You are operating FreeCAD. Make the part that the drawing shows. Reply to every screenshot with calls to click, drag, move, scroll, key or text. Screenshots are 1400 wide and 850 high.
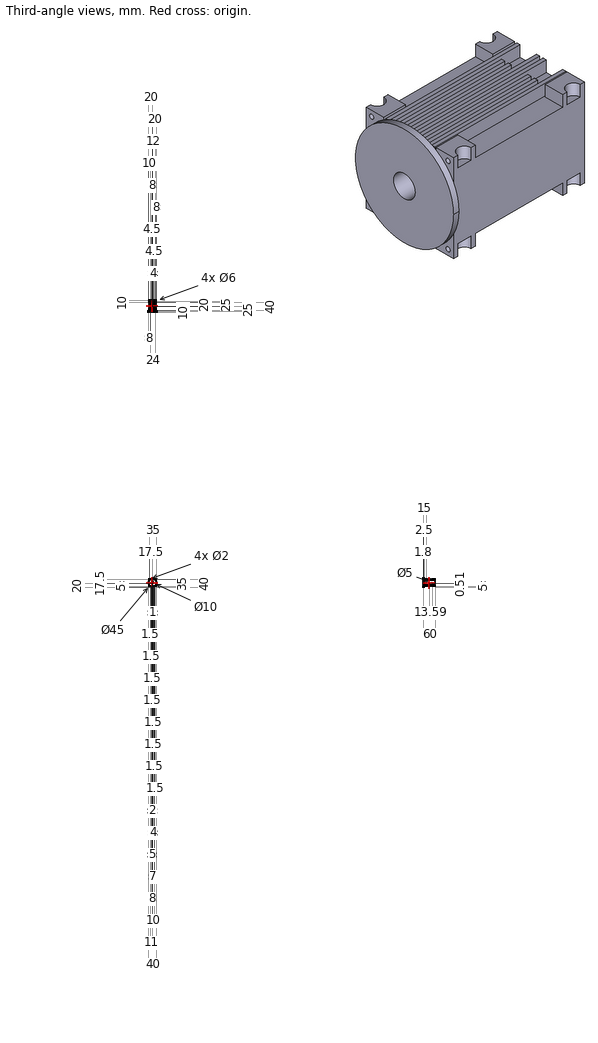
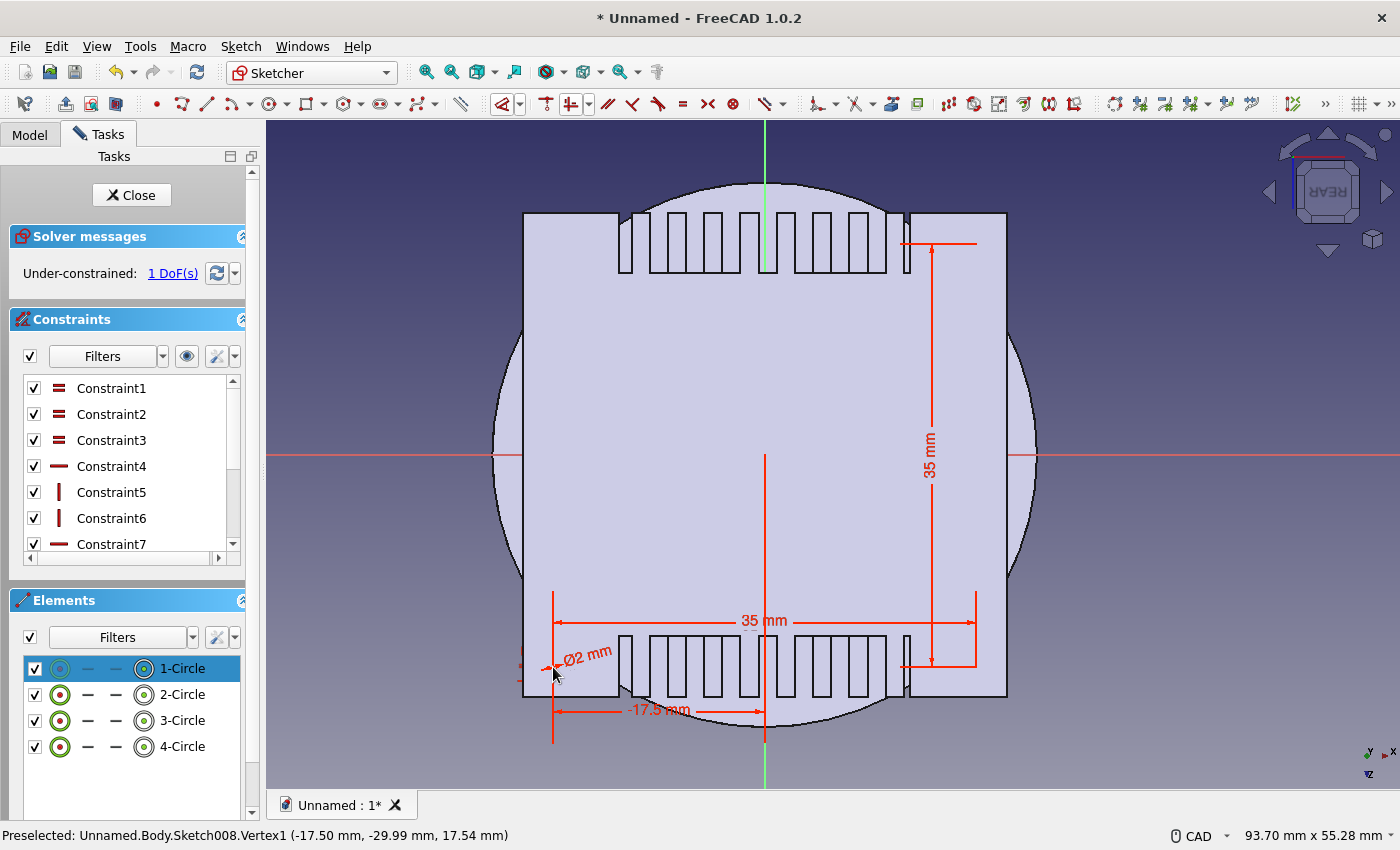
click(520, 104)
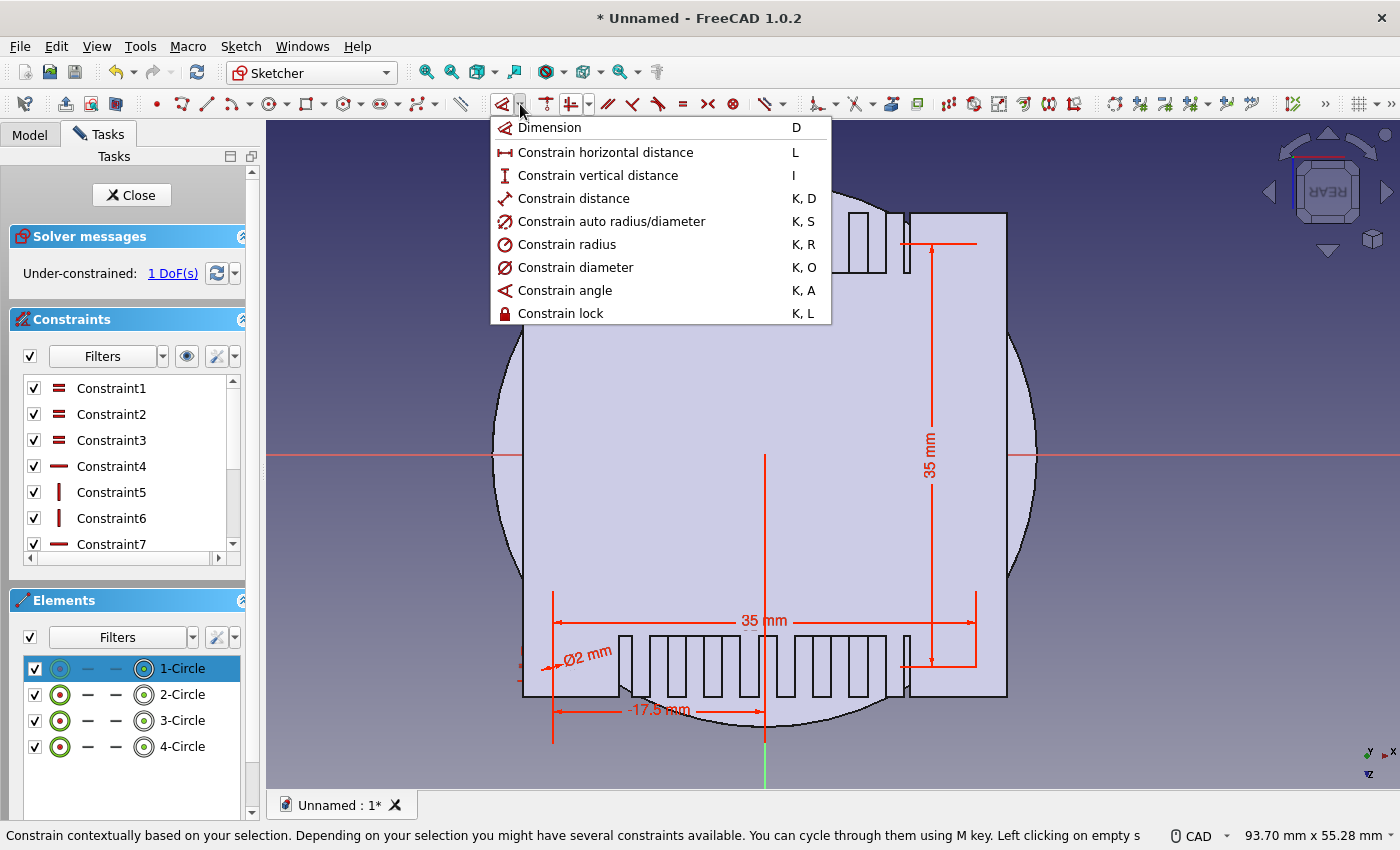
click(661, 176)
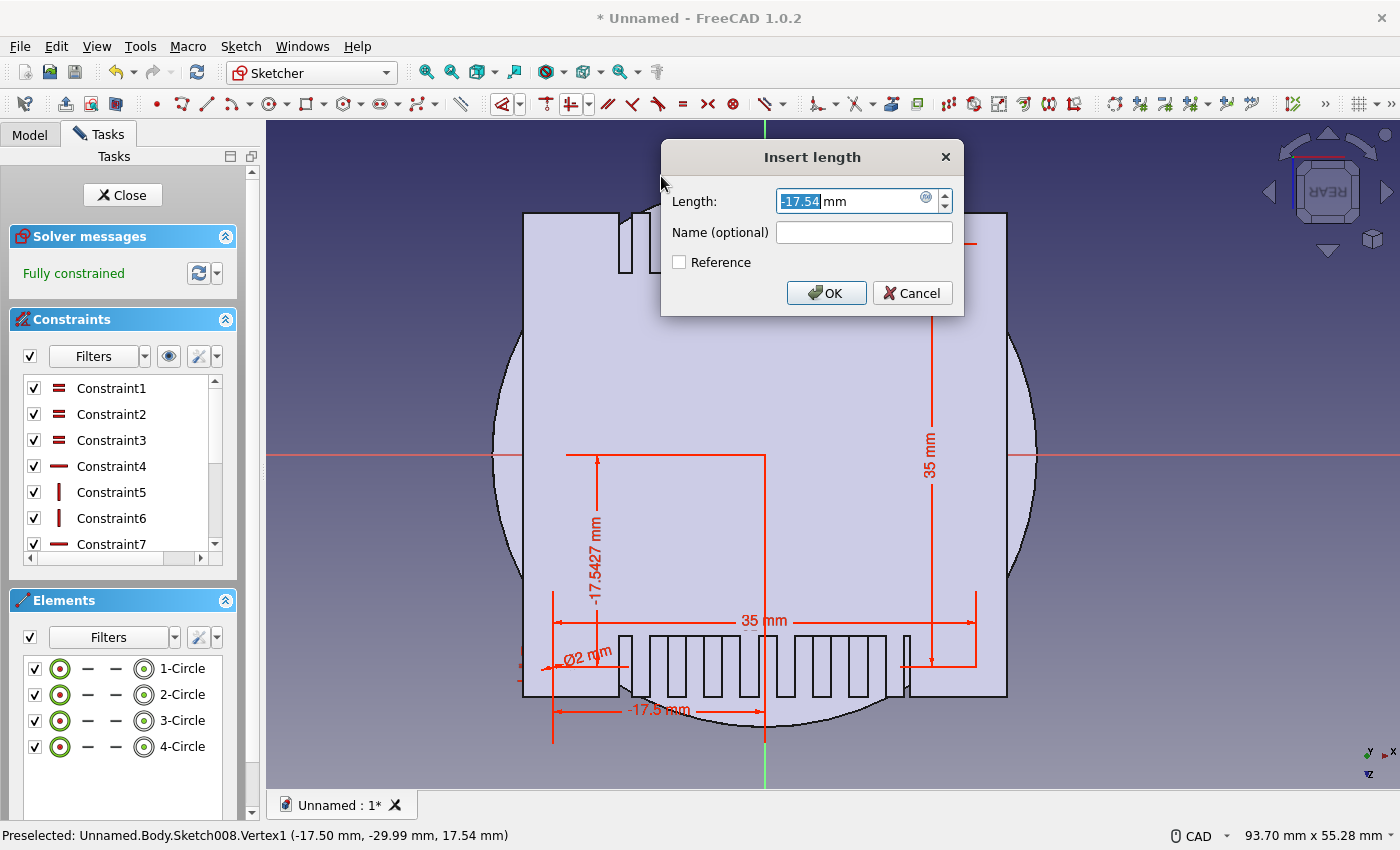
text(-17.5)
key(Return)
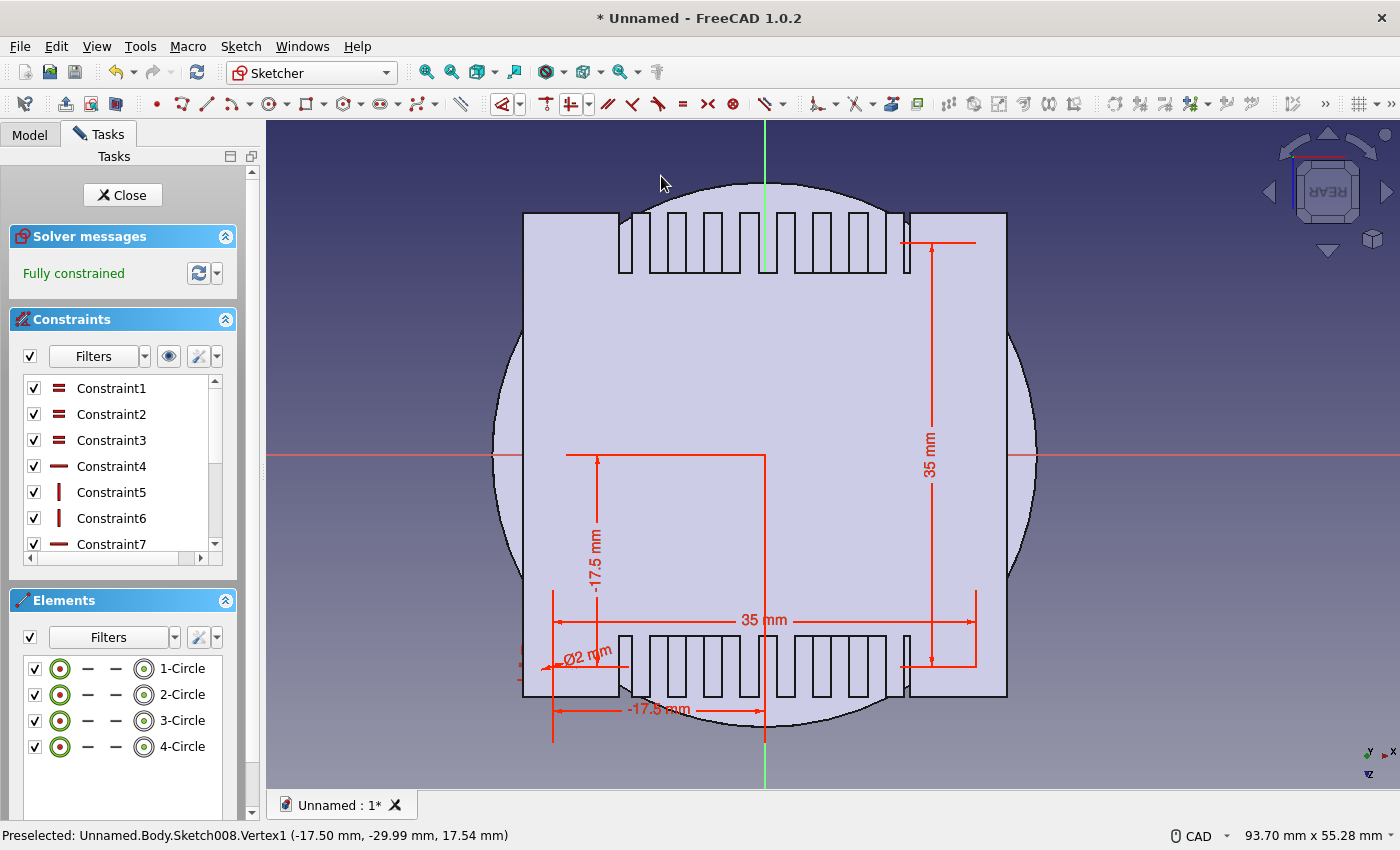
click(123, 195)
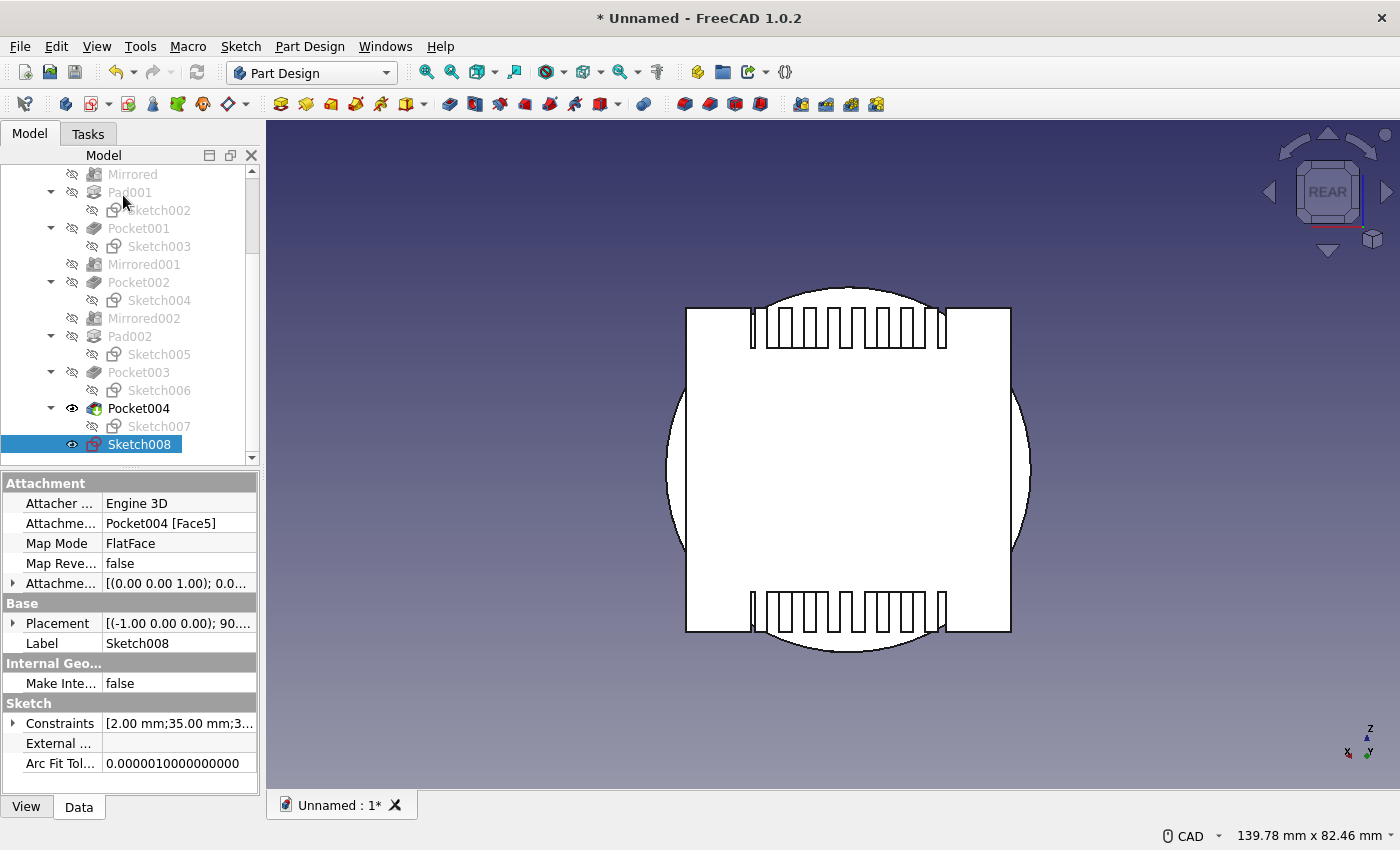
click(450, 104)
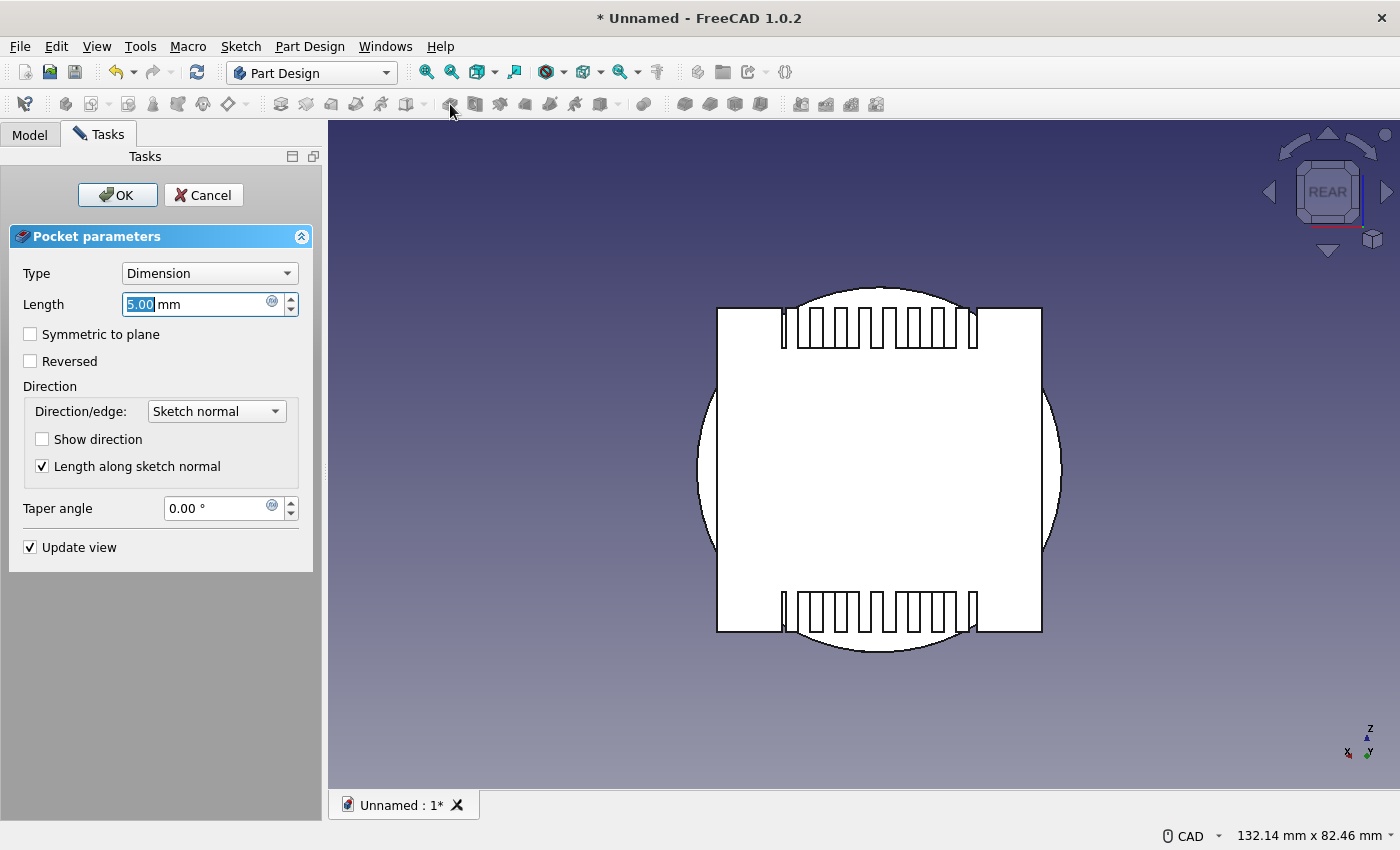
text(1.8)
key(Tab)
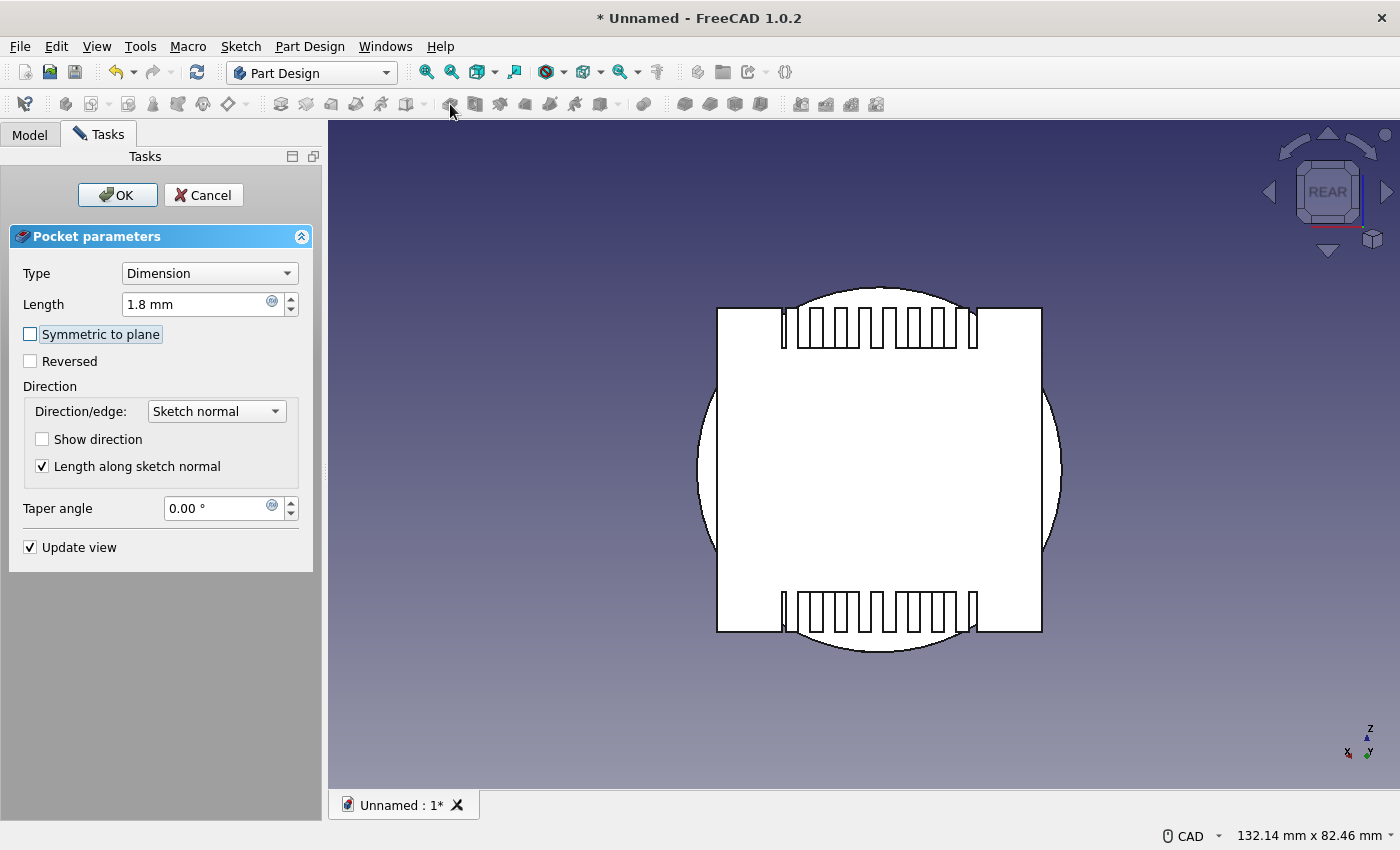
click(31, 361)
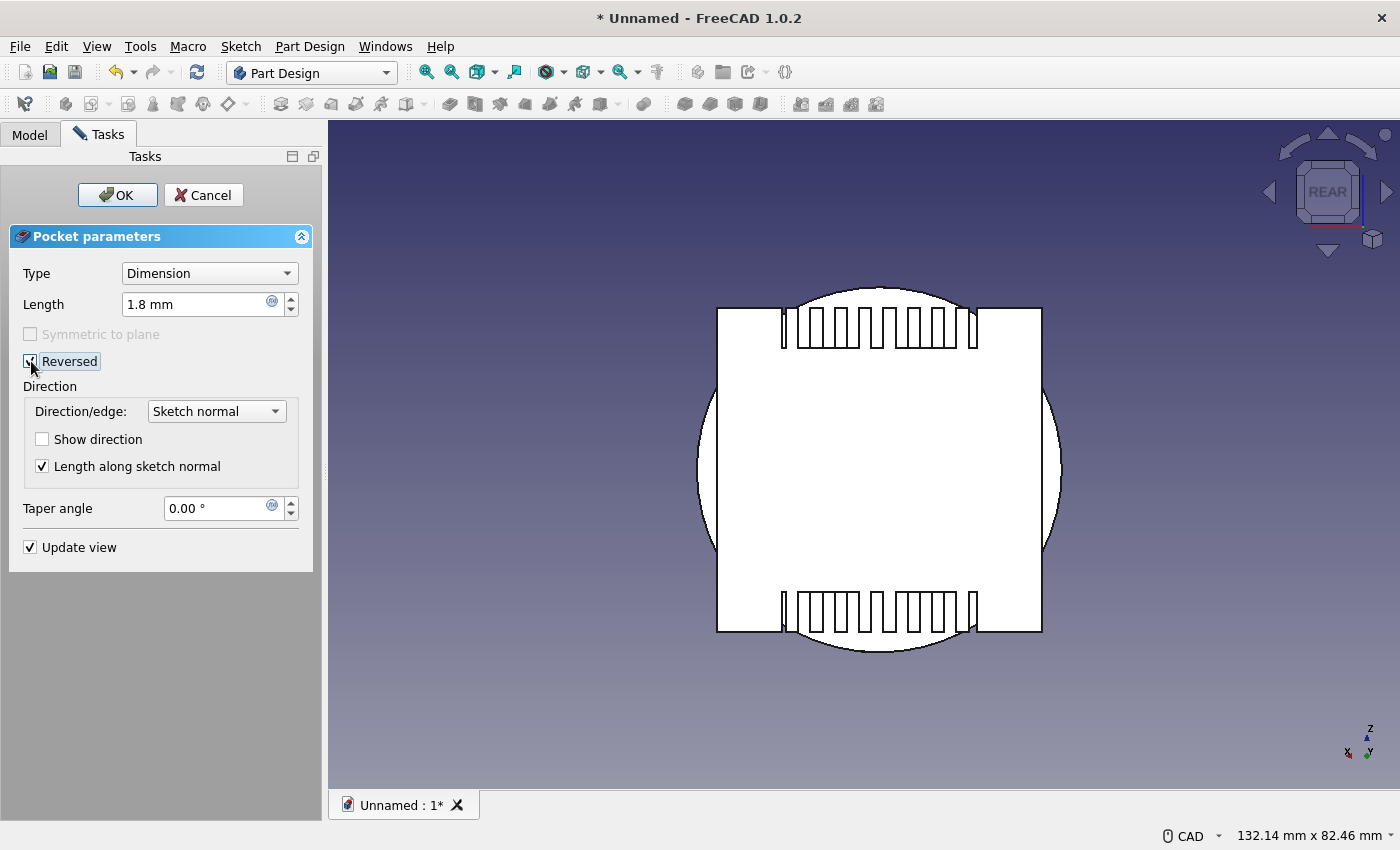
click(118, 195)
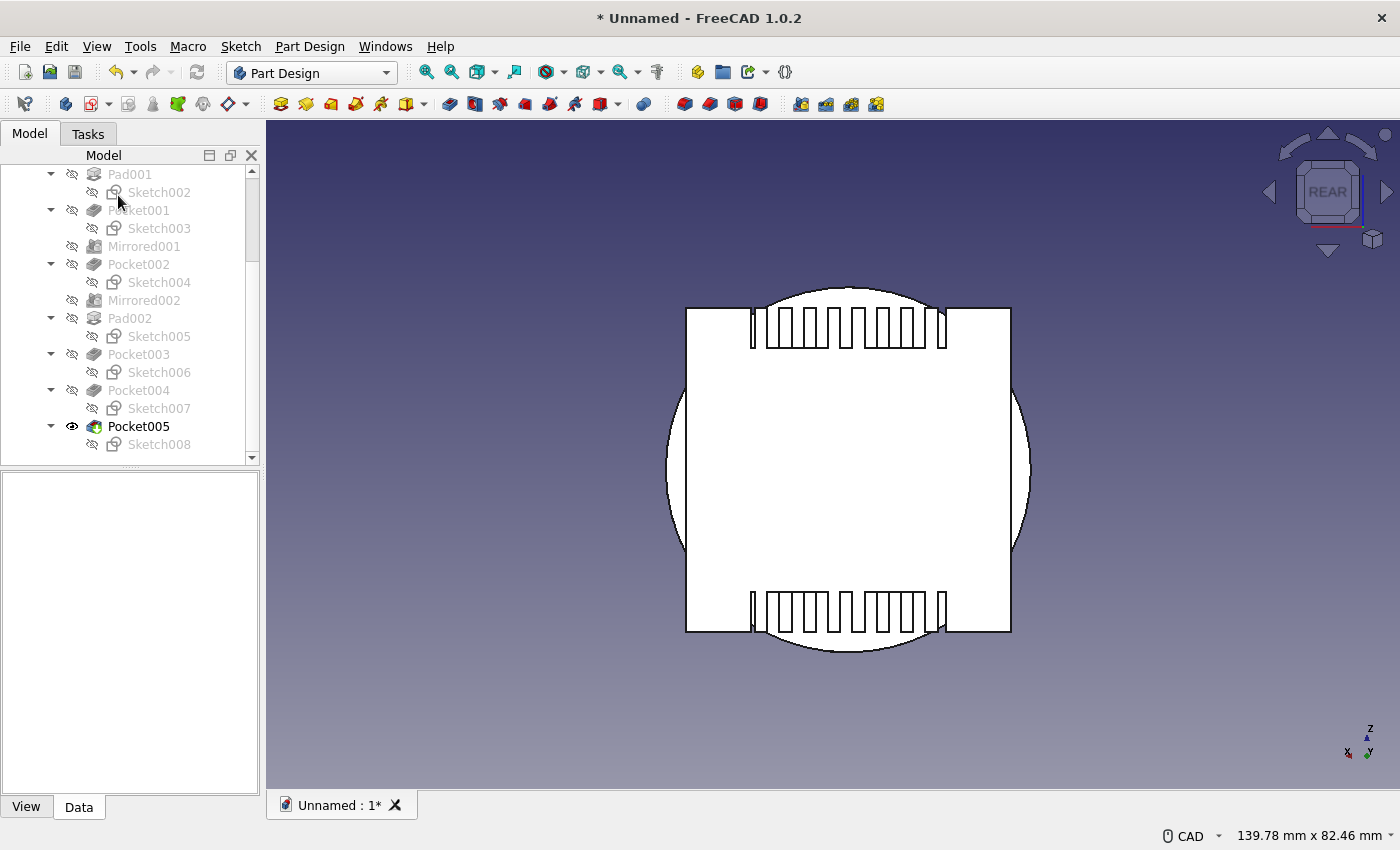
key(0)